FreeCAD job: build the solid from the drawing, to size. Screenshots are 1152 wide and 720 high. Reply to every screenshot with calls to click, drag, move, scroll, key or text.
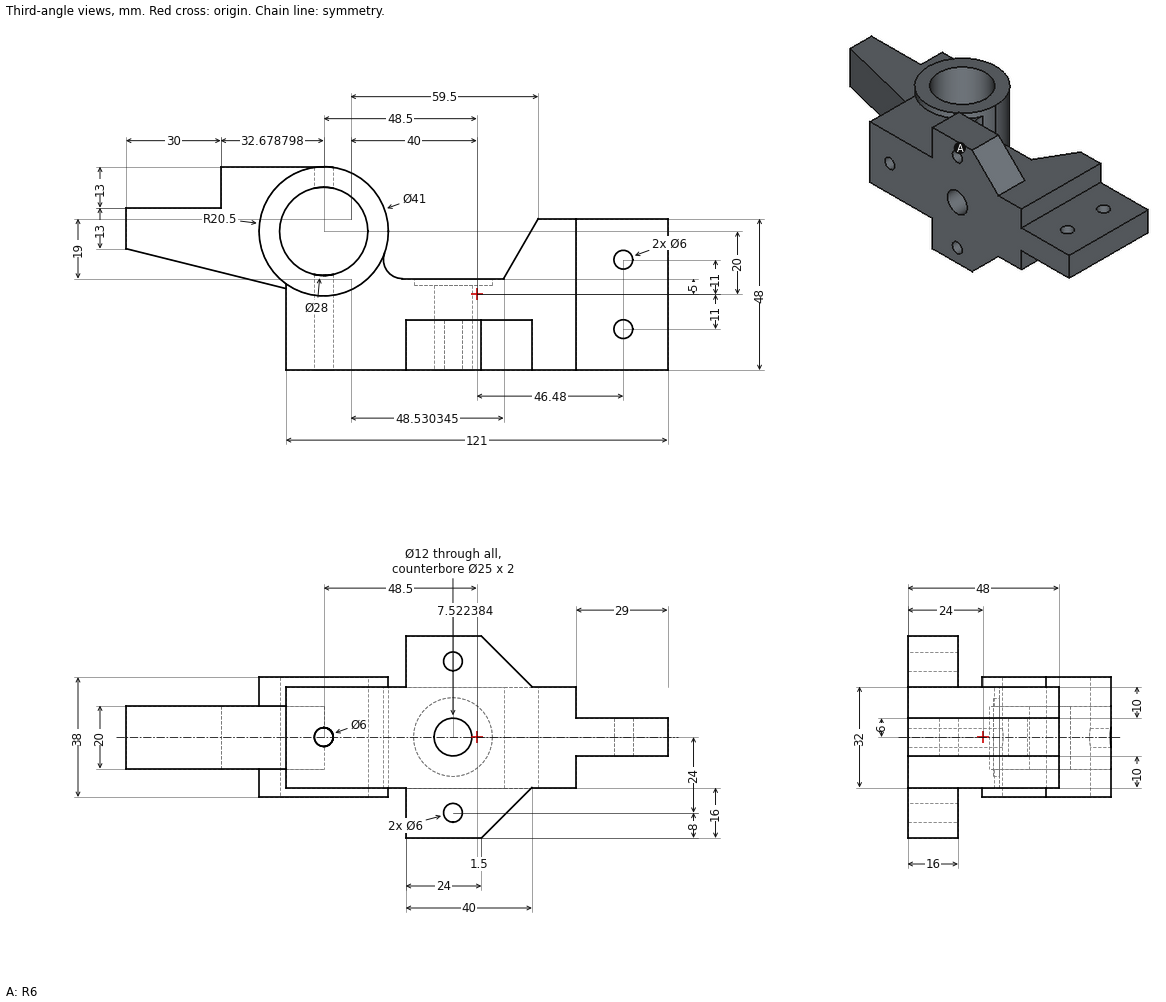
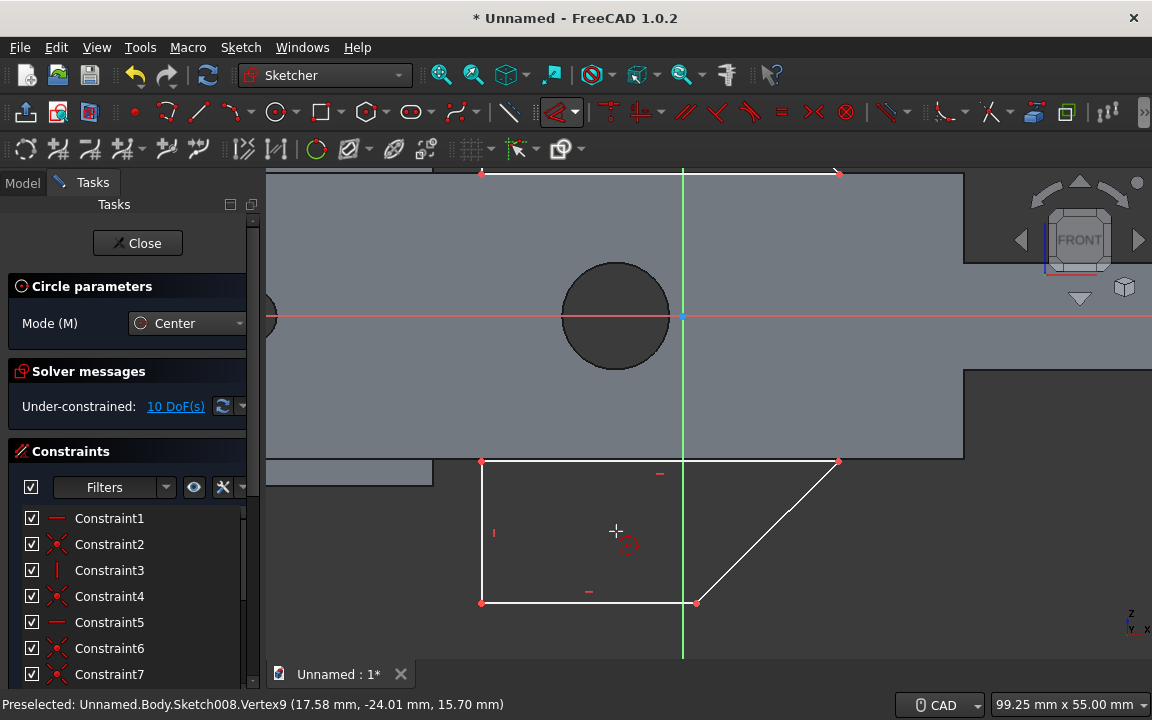
click(616, 530)
move(635, 511)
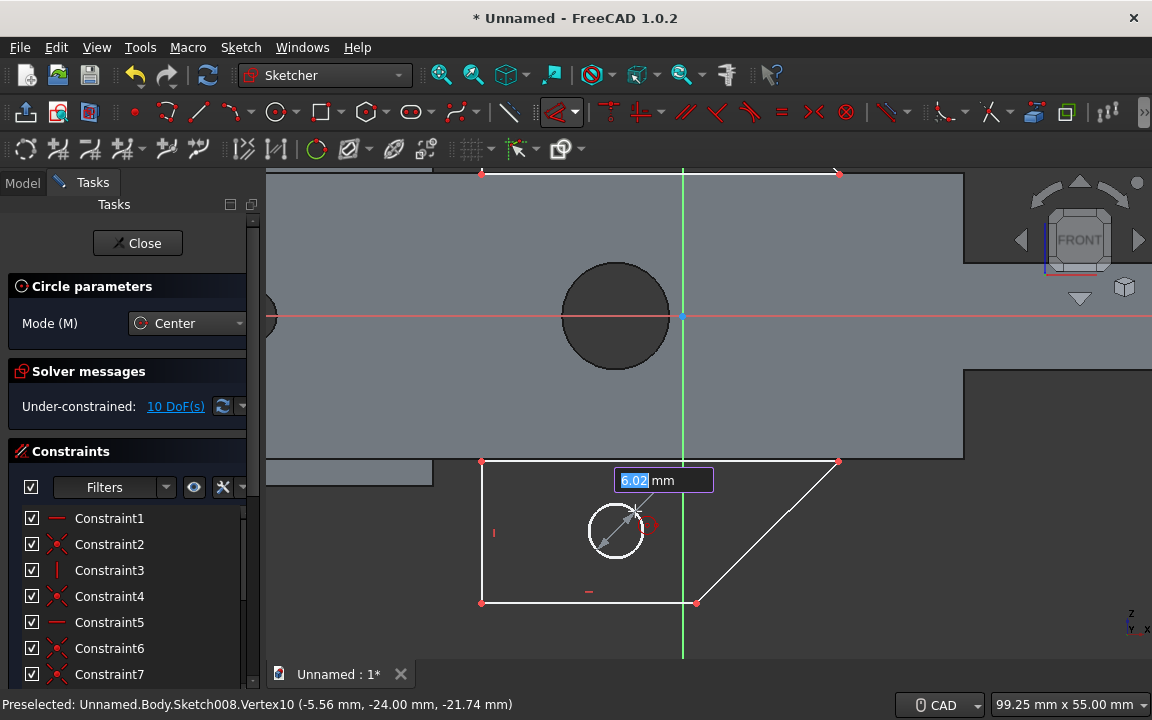
text(6)
key(Return)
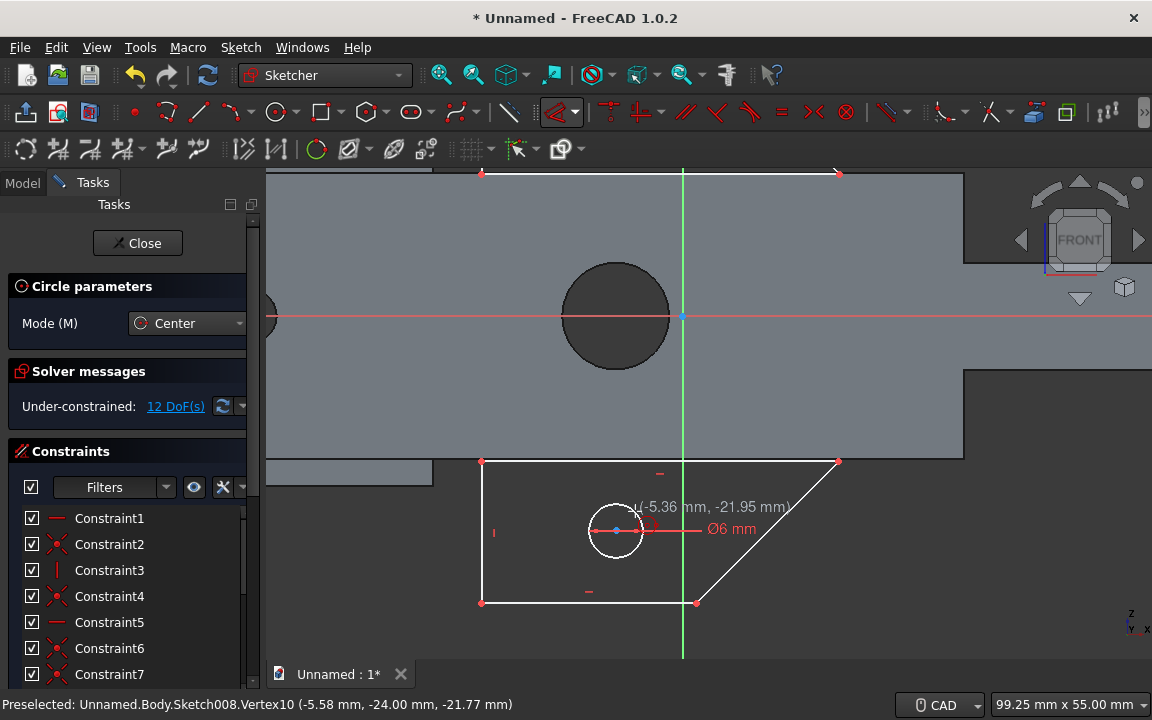
scroll(616, 532, down, 3)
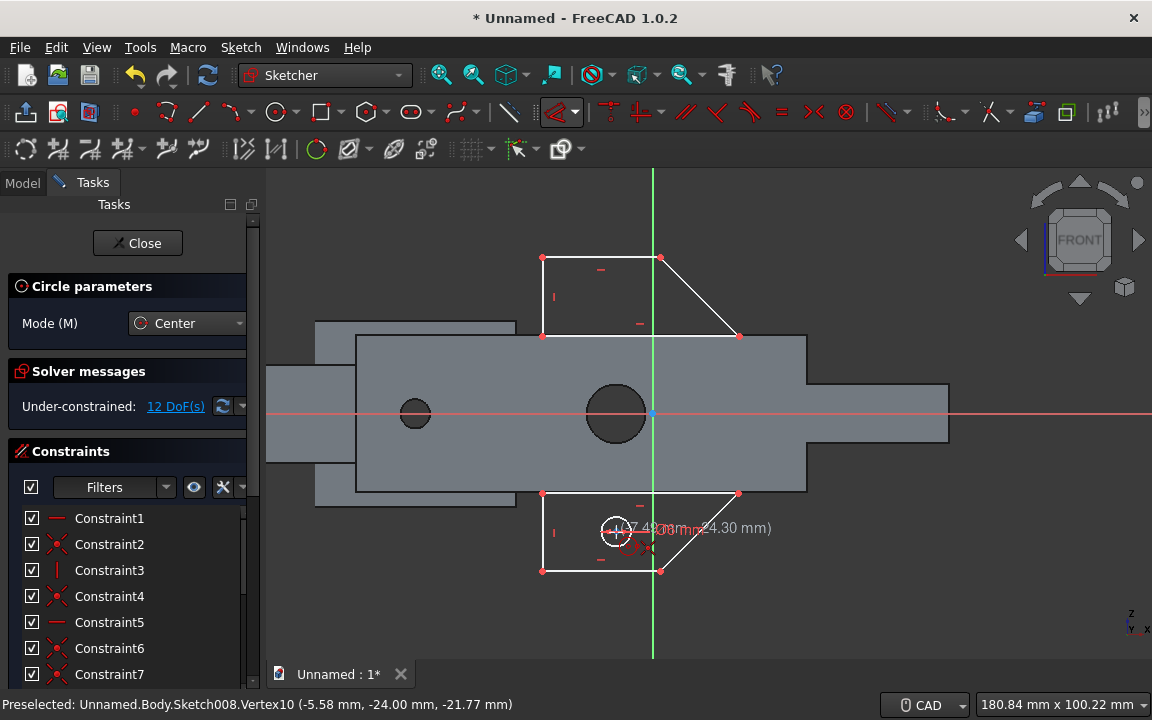
scroll(616, 296, up, 3)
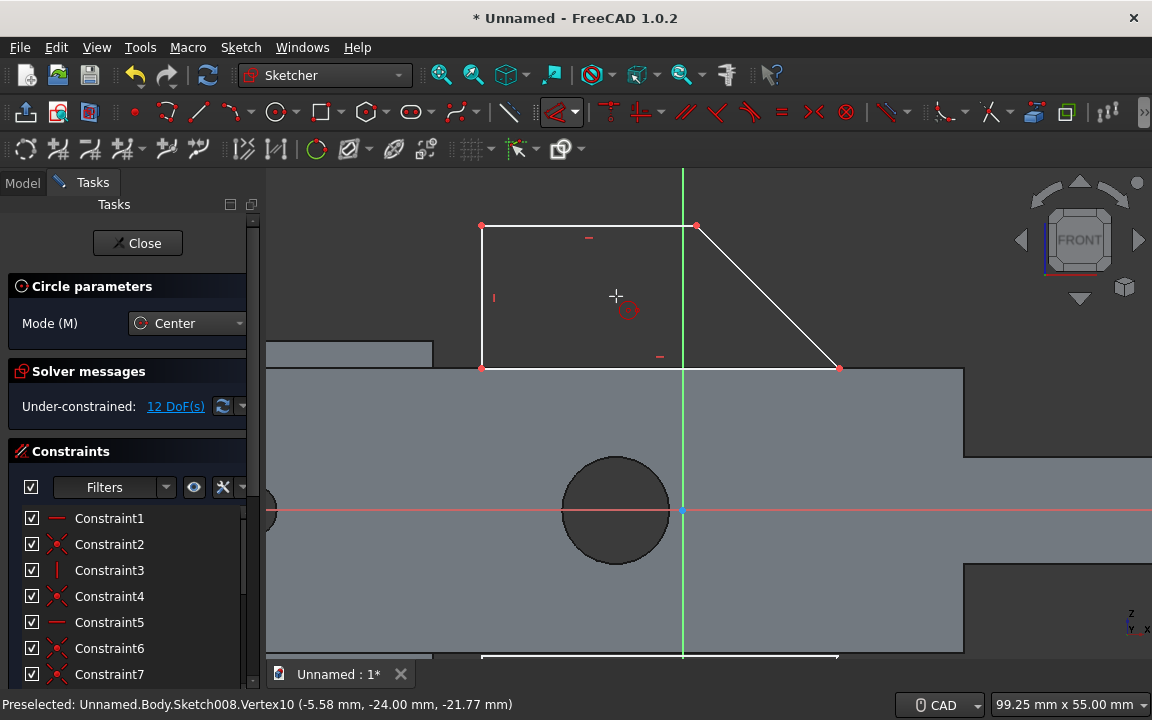
click(616, 296)
move(635, 277)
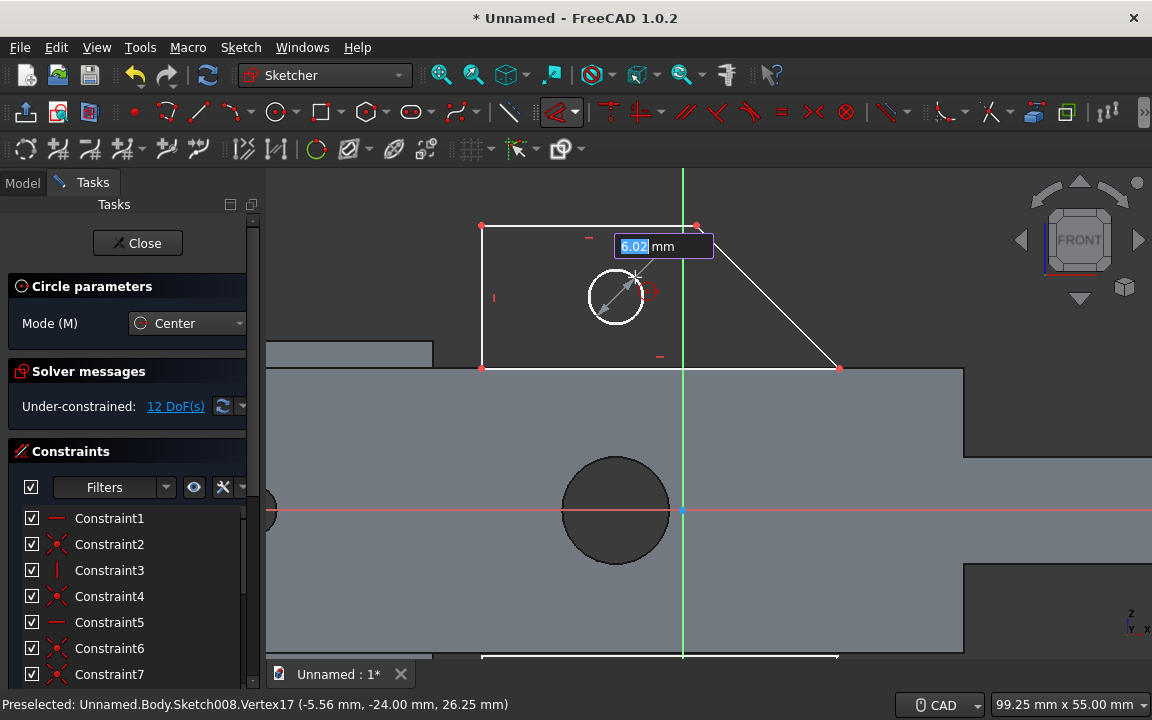
text(6)
key(Return)
key(Escape)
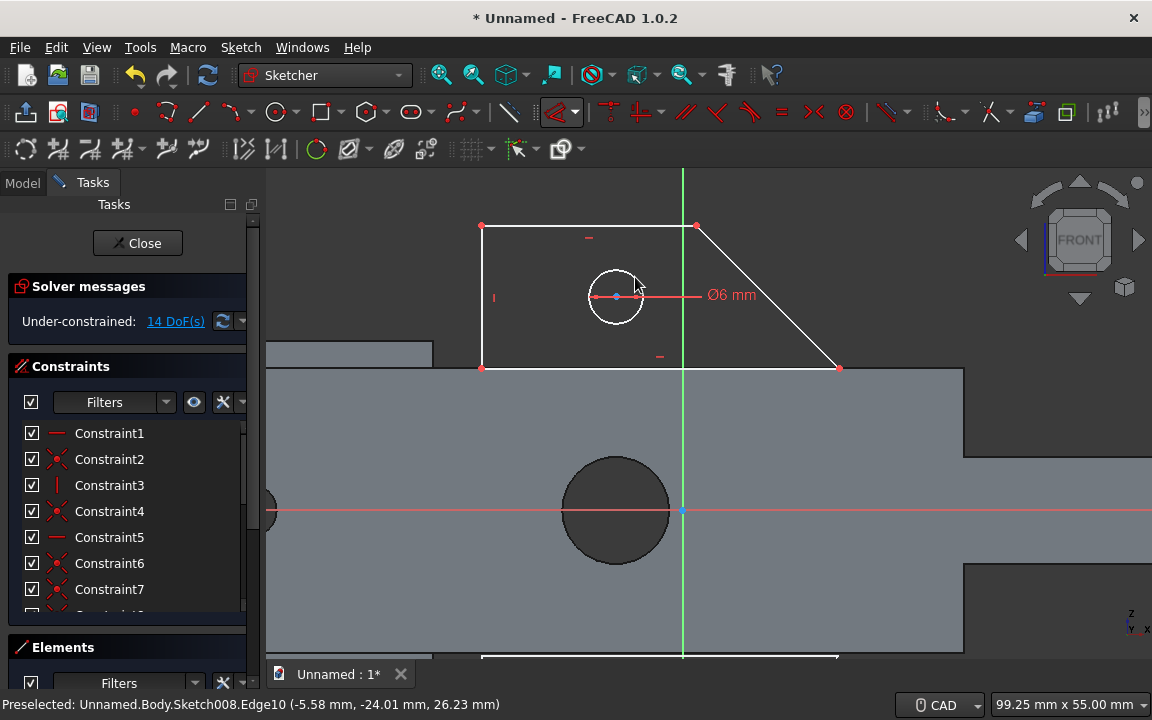
scroll(616, 296, down, 3)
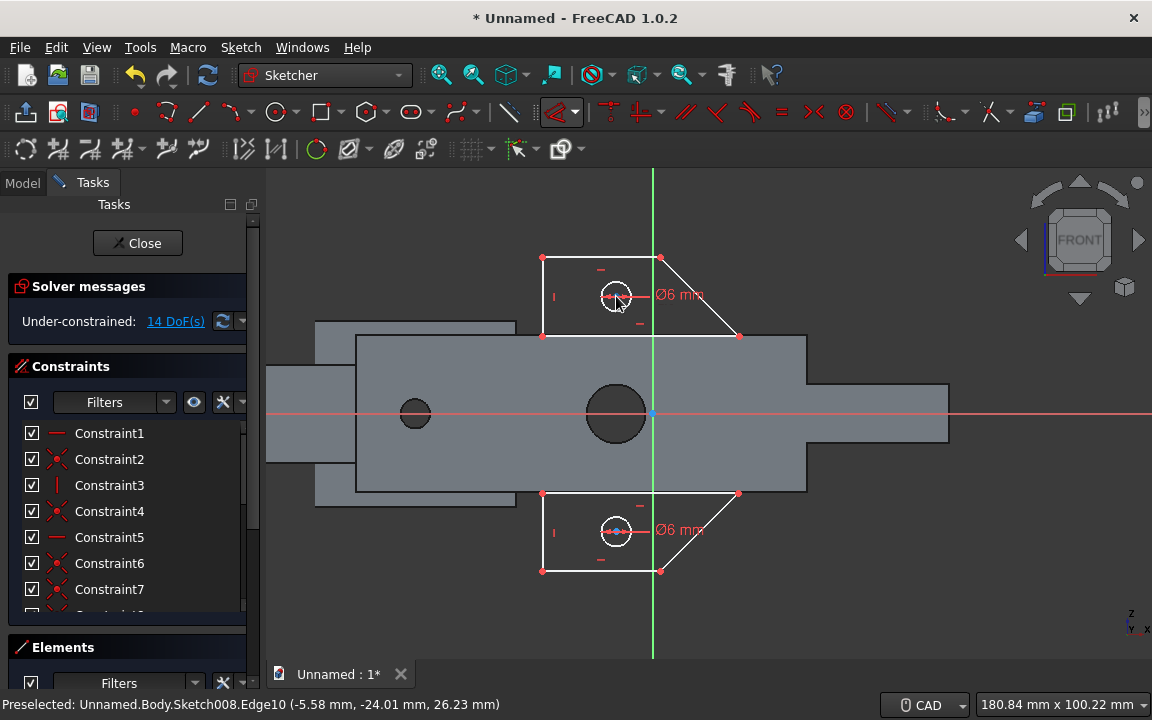
click(616, 532)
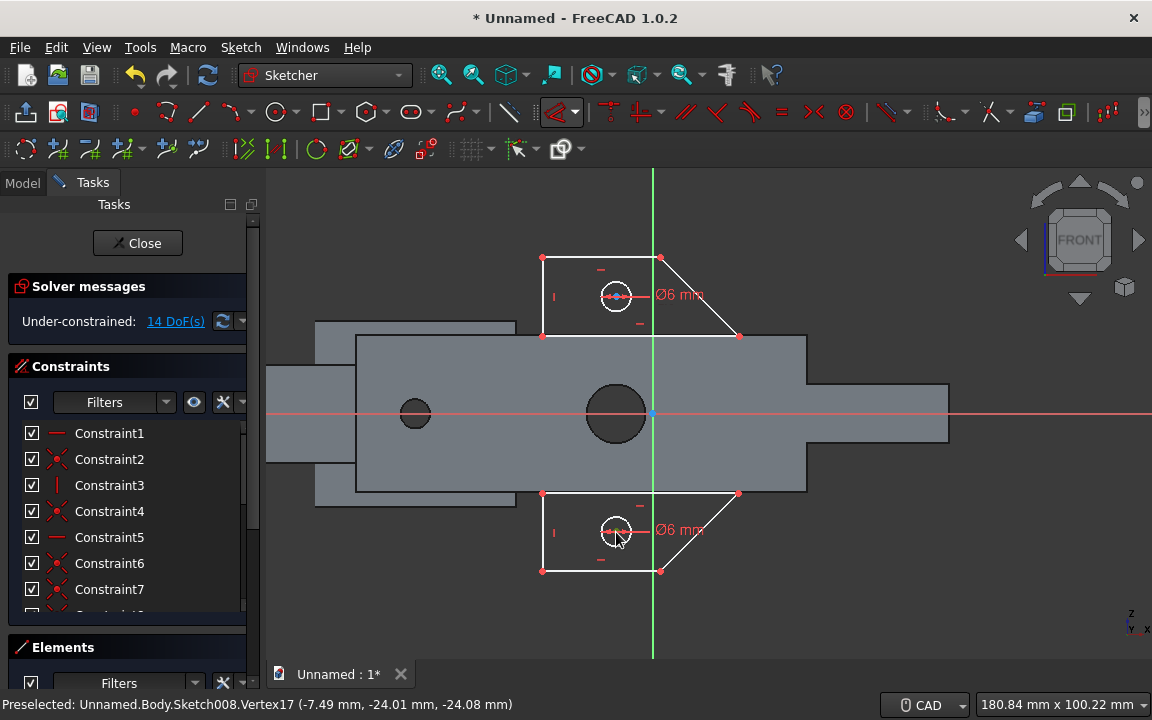
click(616, 297)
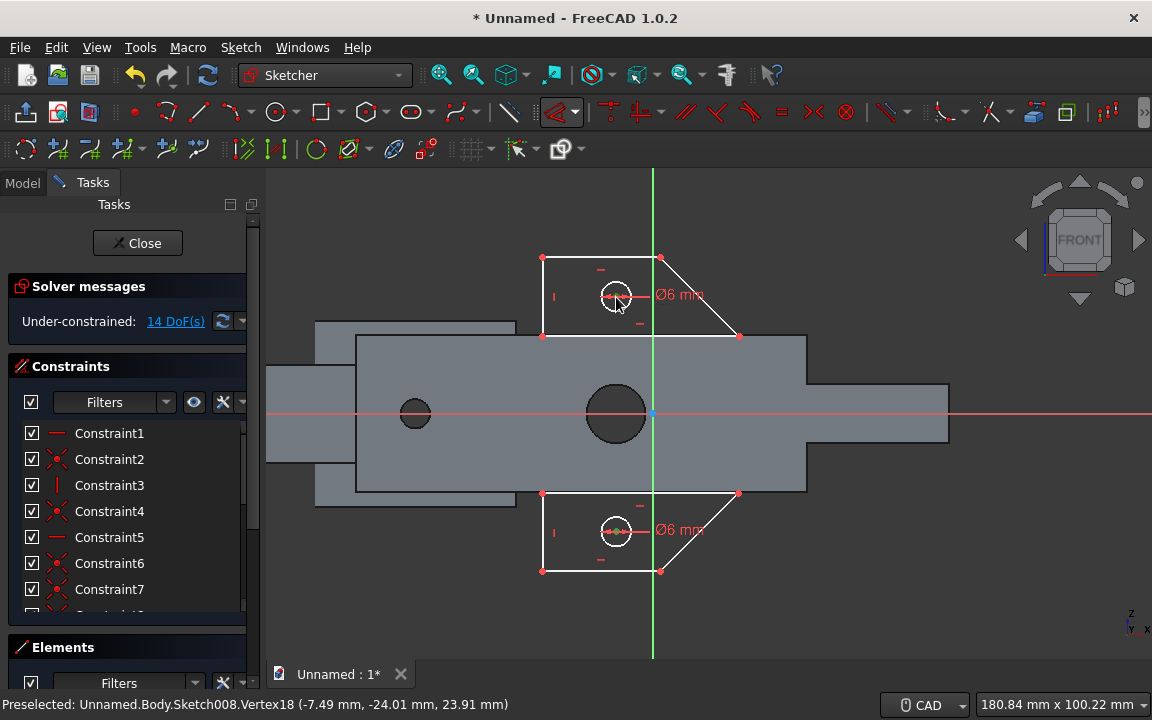
click(344, 414)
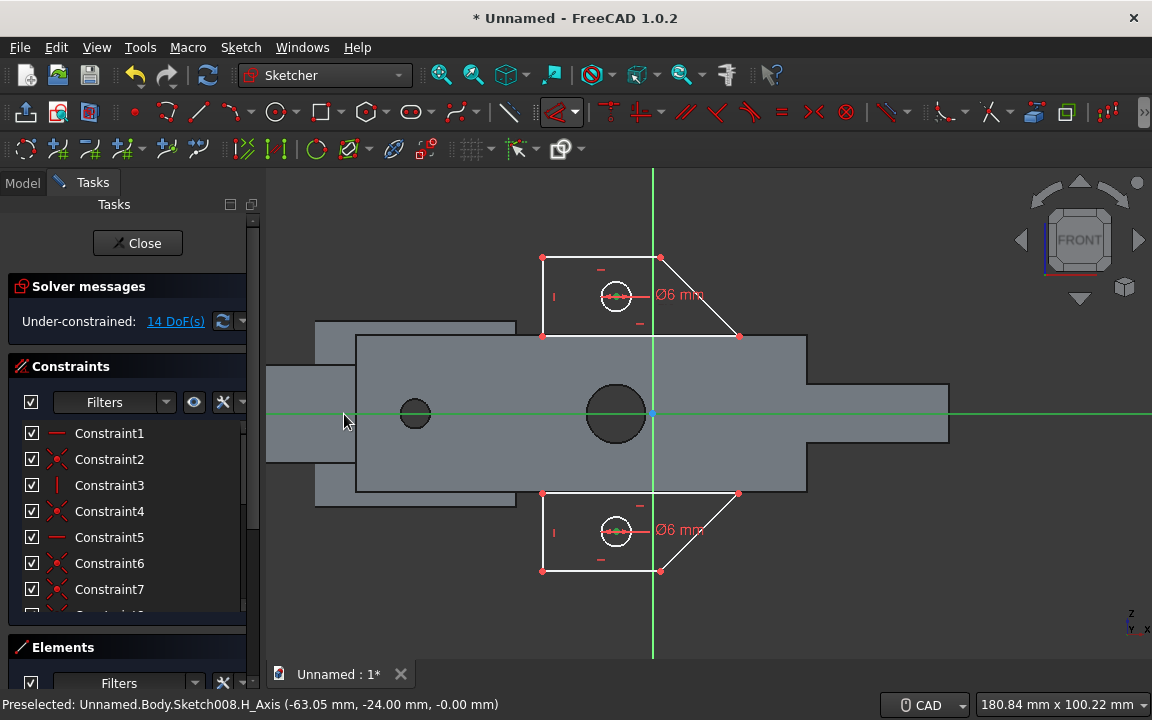
click(814, 112)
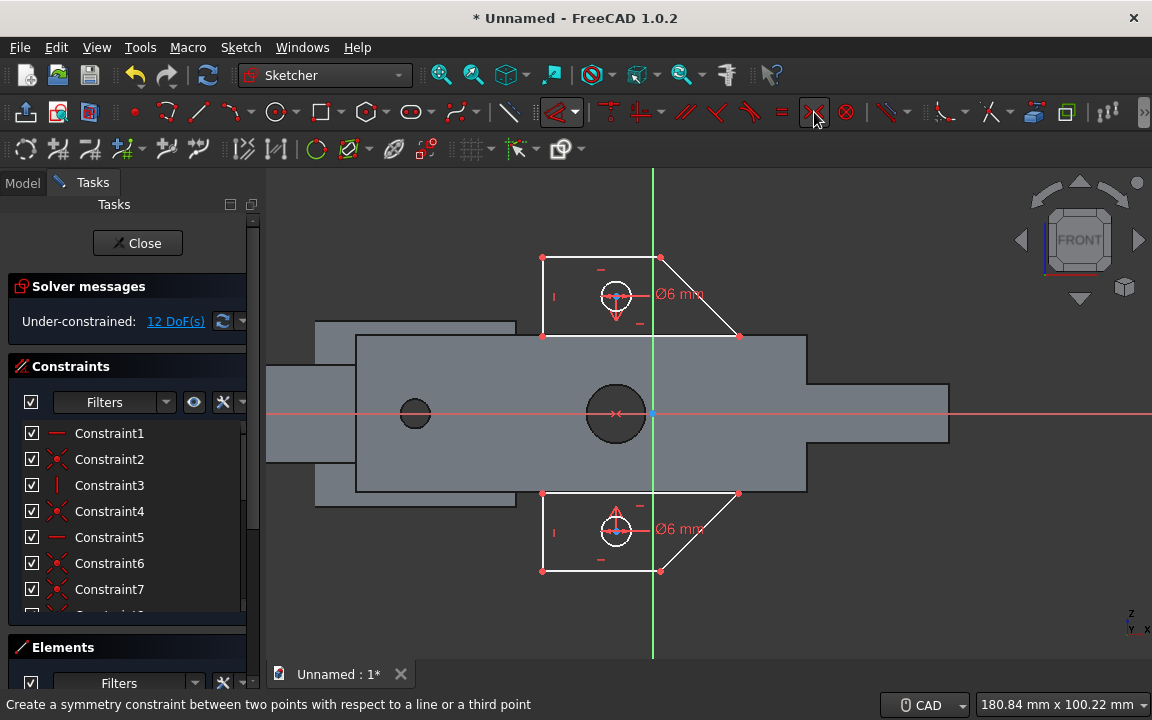
click(739, 493)